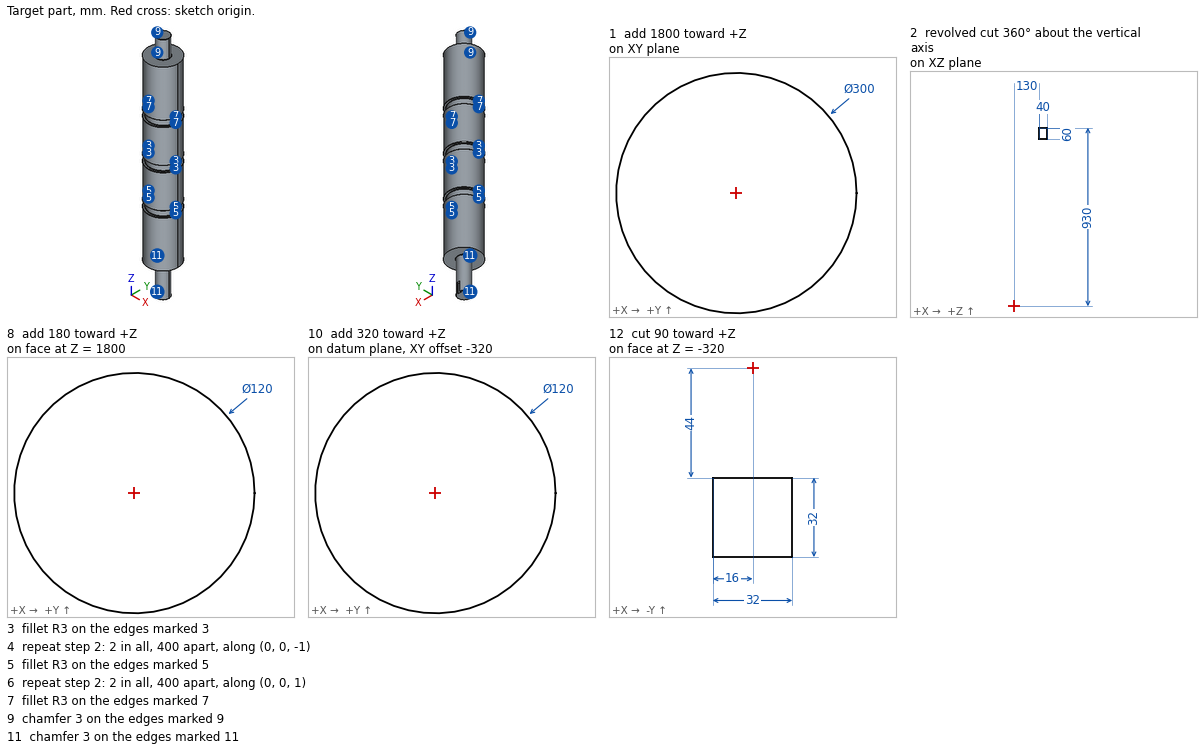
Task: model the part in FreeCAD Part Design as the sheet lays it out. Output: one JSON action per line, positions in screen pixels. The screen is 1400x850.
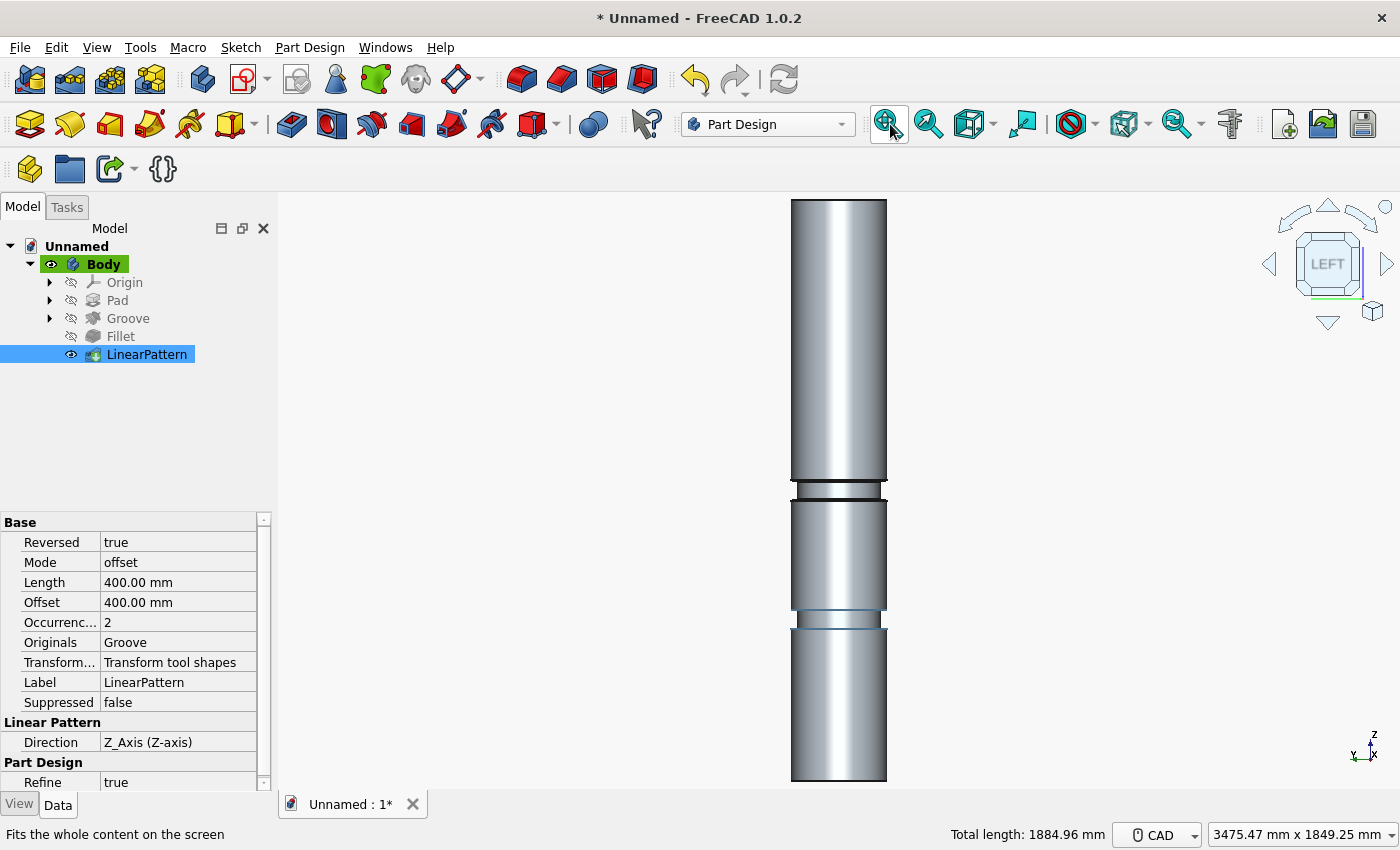
{"action": "key", "text": "v 3"}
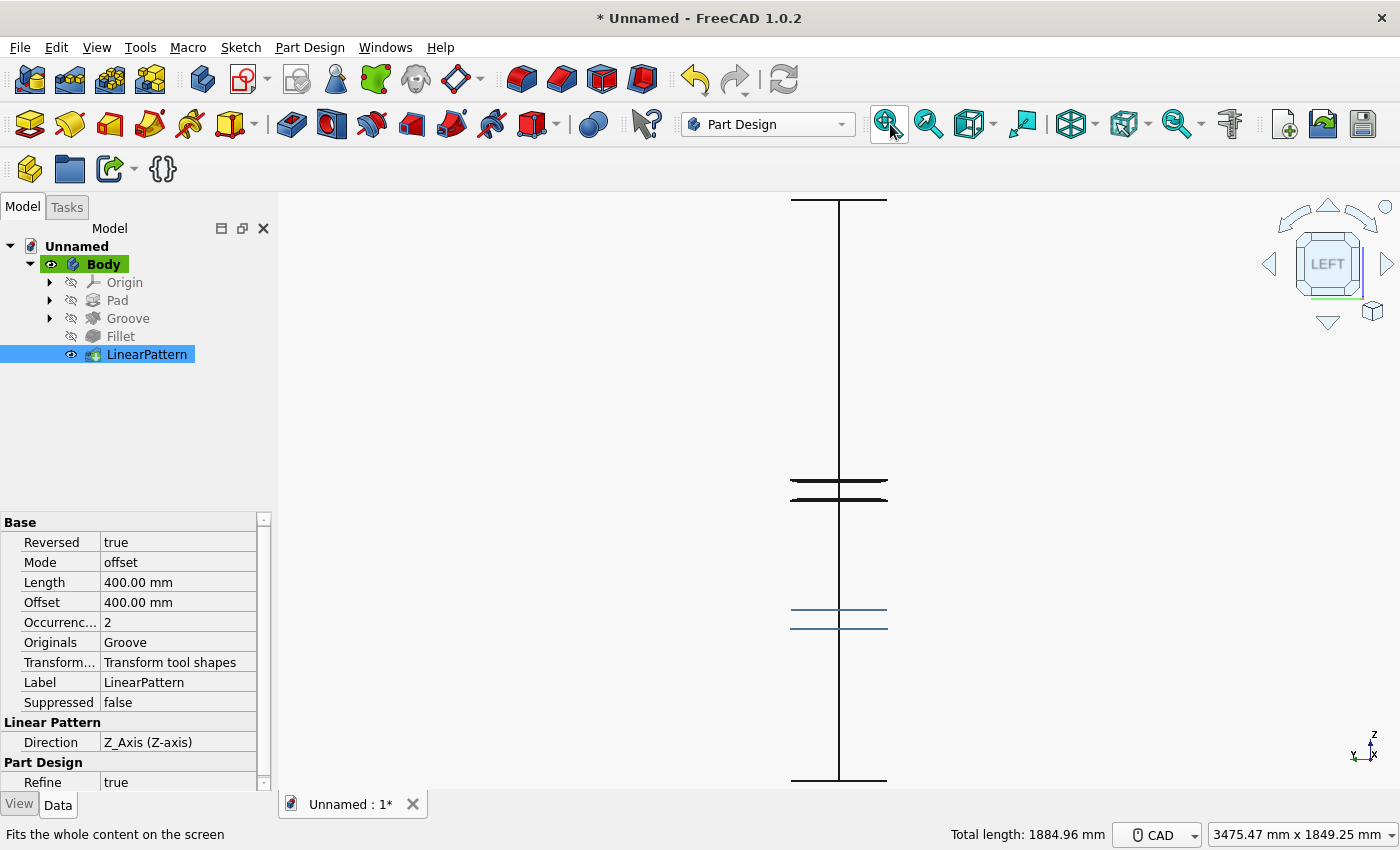
{"action": "key", "text": "0"}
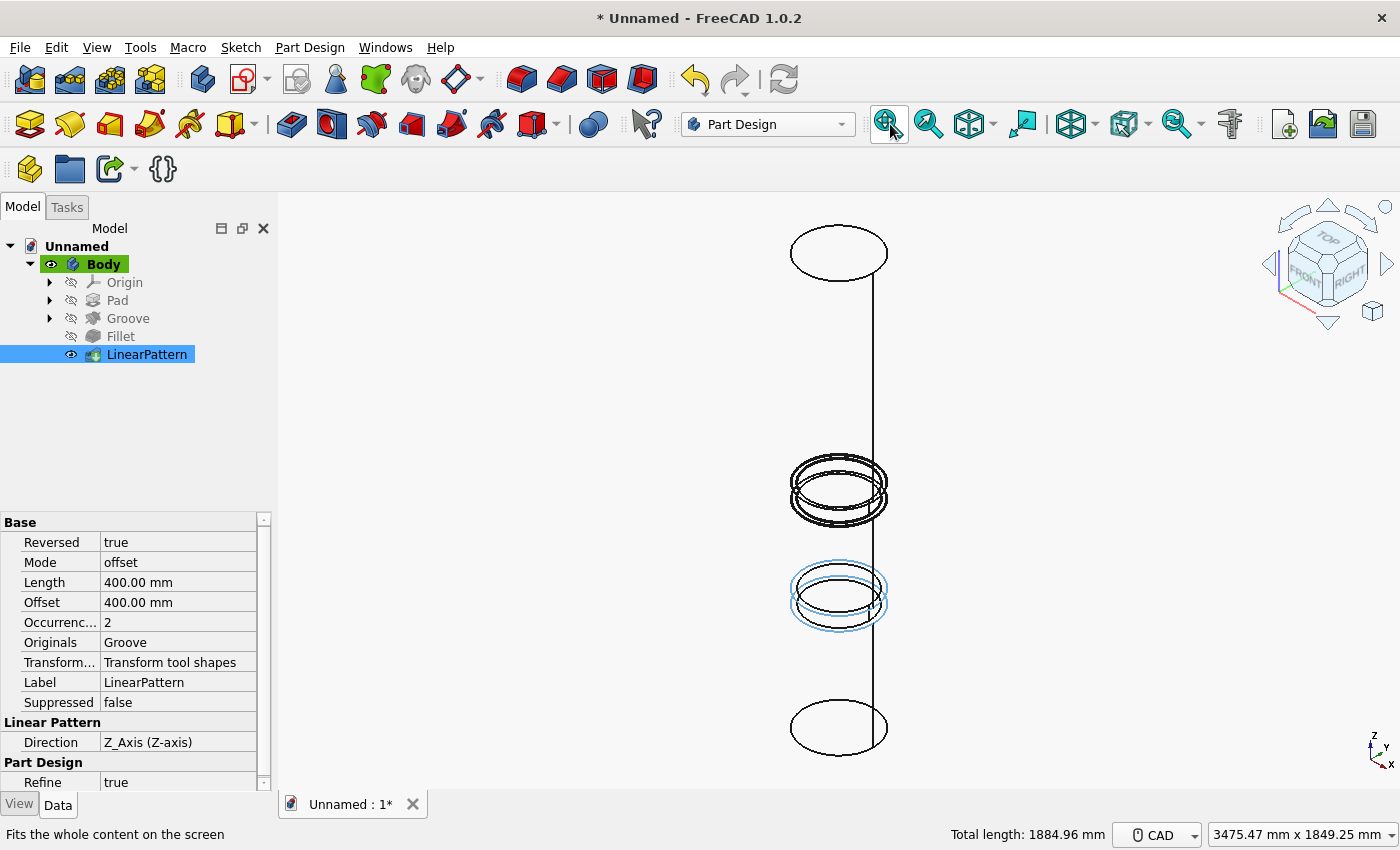
{"action": "left_click", "coordinate": [809, 570], "text": "ctrl"}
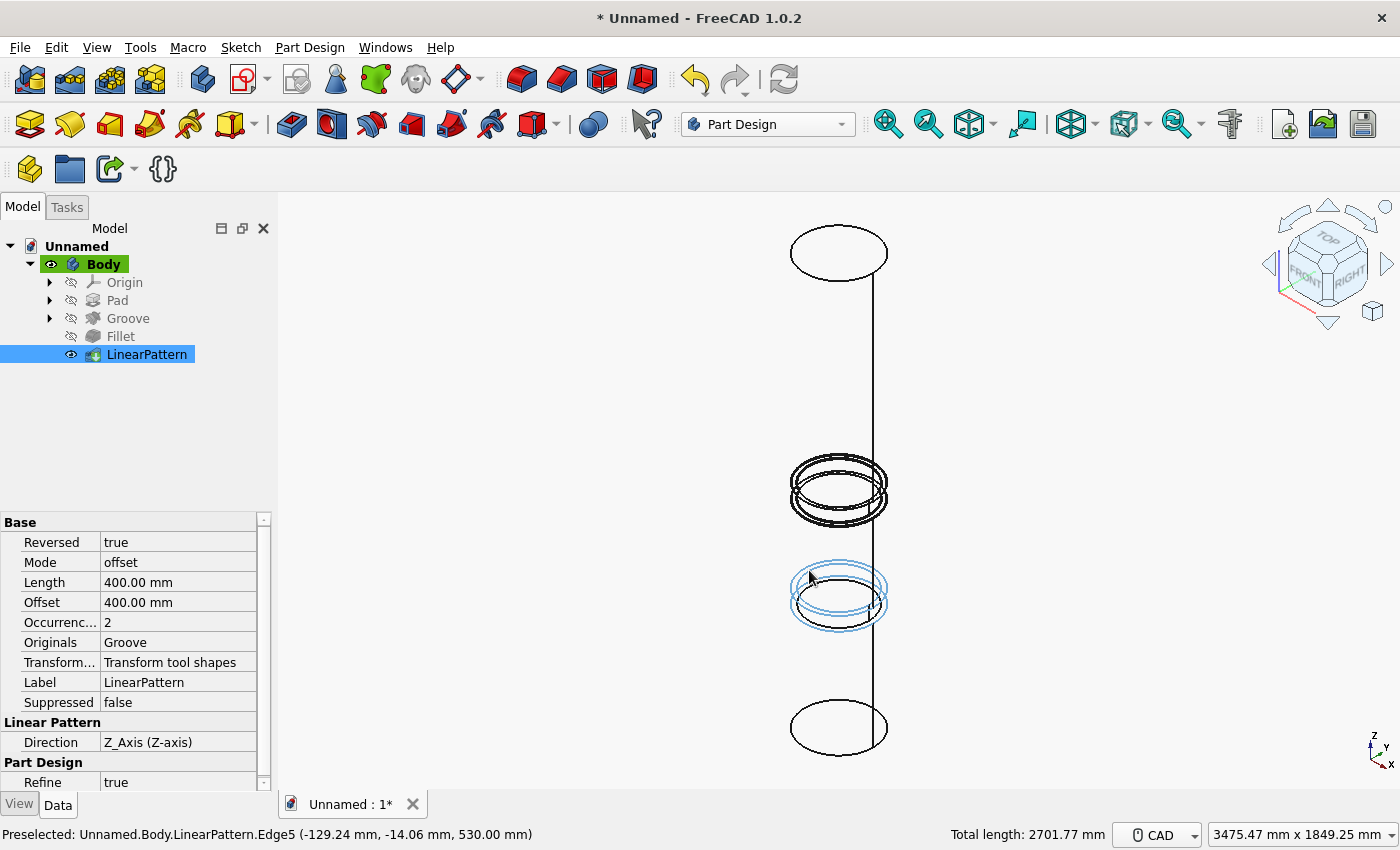
{"action": "left_click", "coordinate": [809, 586], "text": "ctrl"}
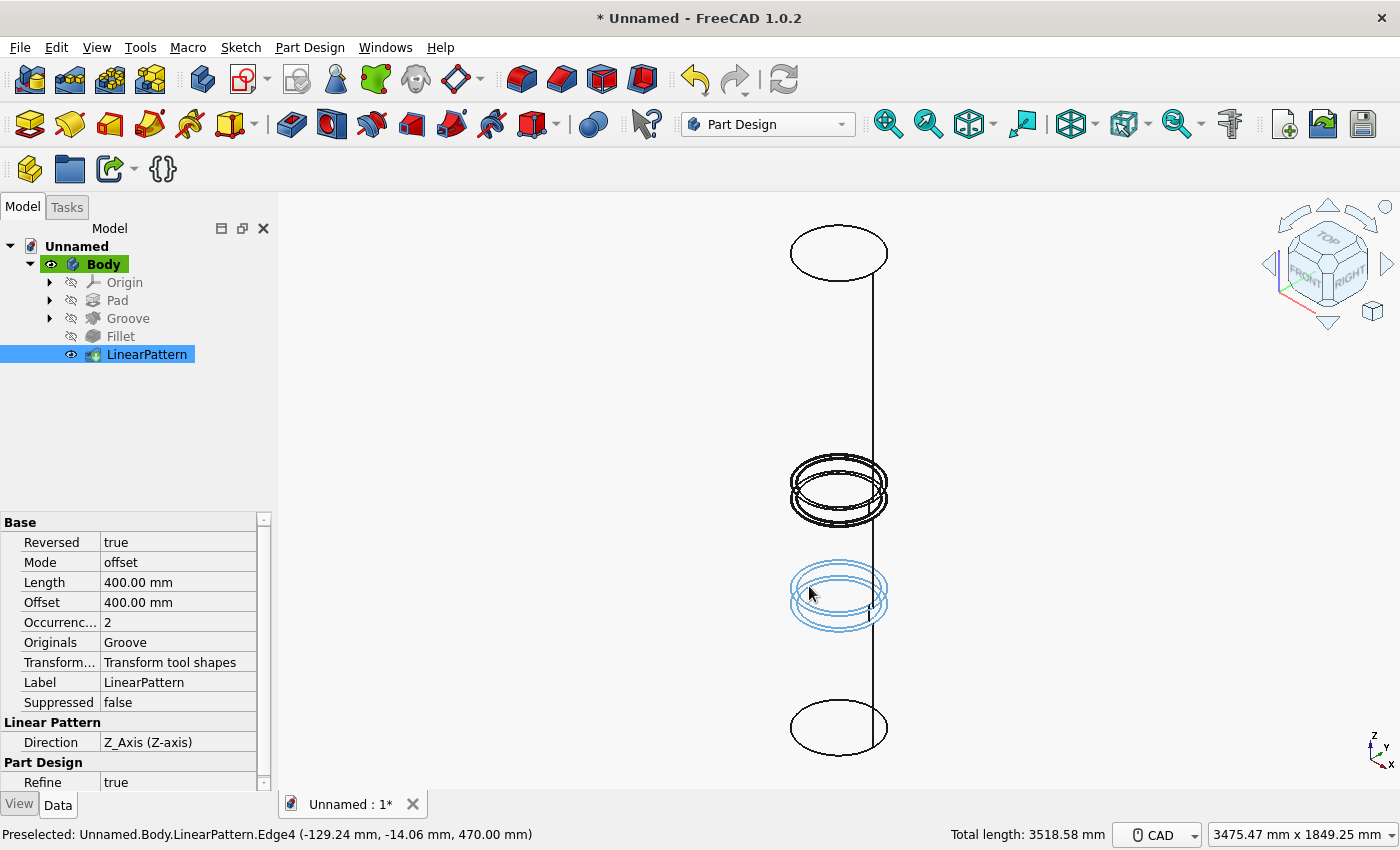
{"action": "key", "text": "v 1"}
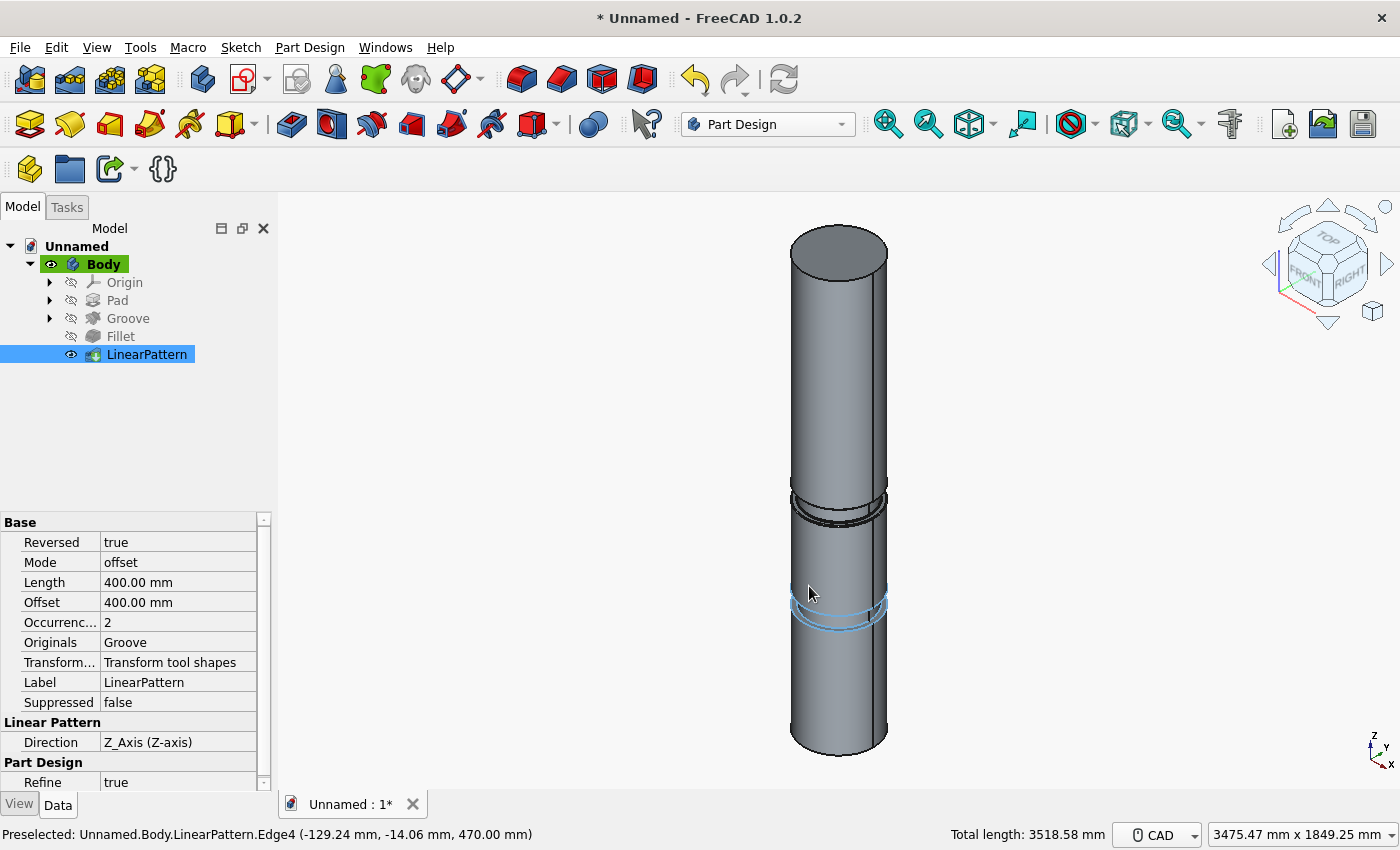
{"action": "left_click", "coordinate": [522, 80]}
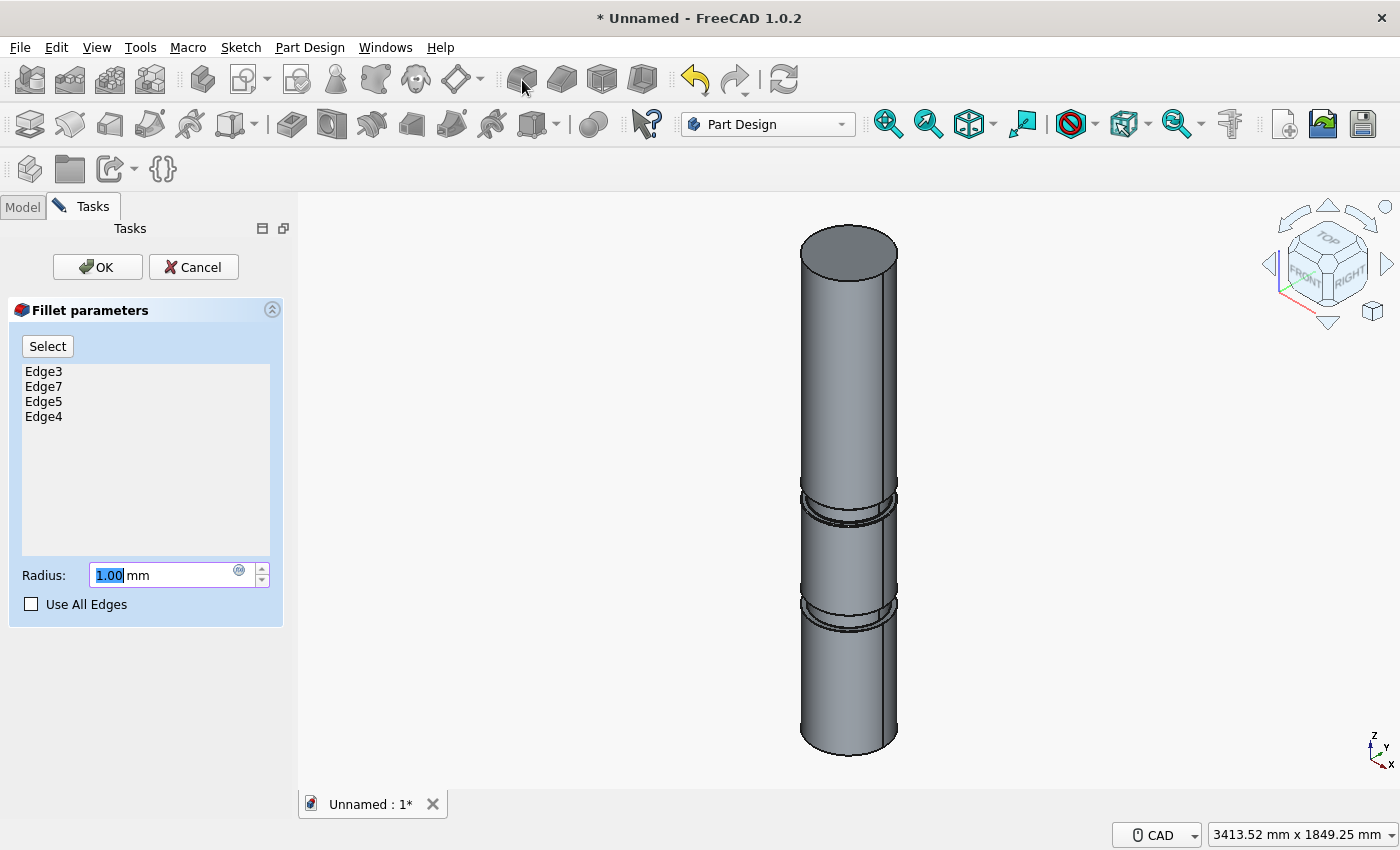
{"action": "type", "text": "3"}
{"action": "key", "text": "Tab"}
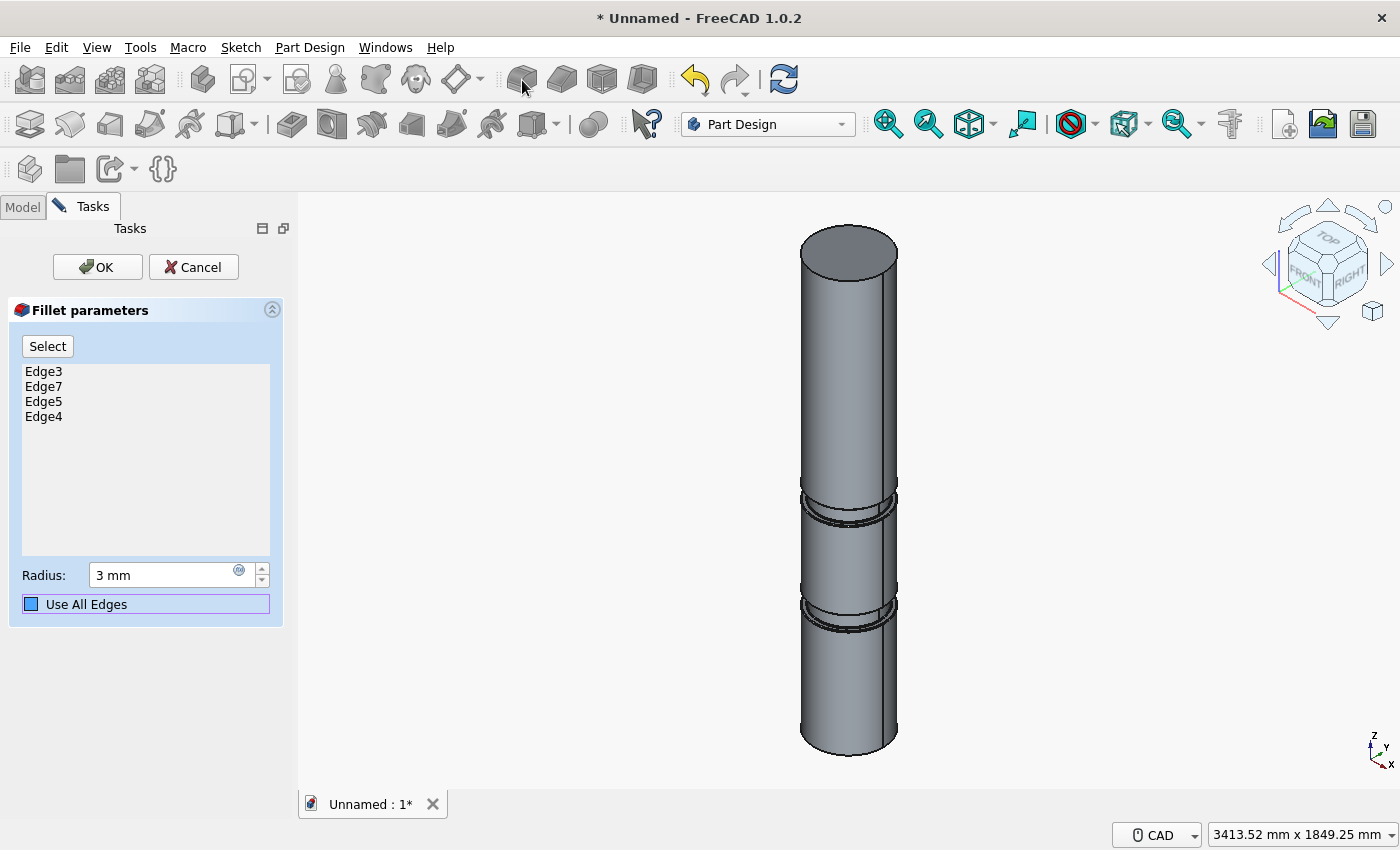
{"action": "left_click", "coordinate": [98, 267]}